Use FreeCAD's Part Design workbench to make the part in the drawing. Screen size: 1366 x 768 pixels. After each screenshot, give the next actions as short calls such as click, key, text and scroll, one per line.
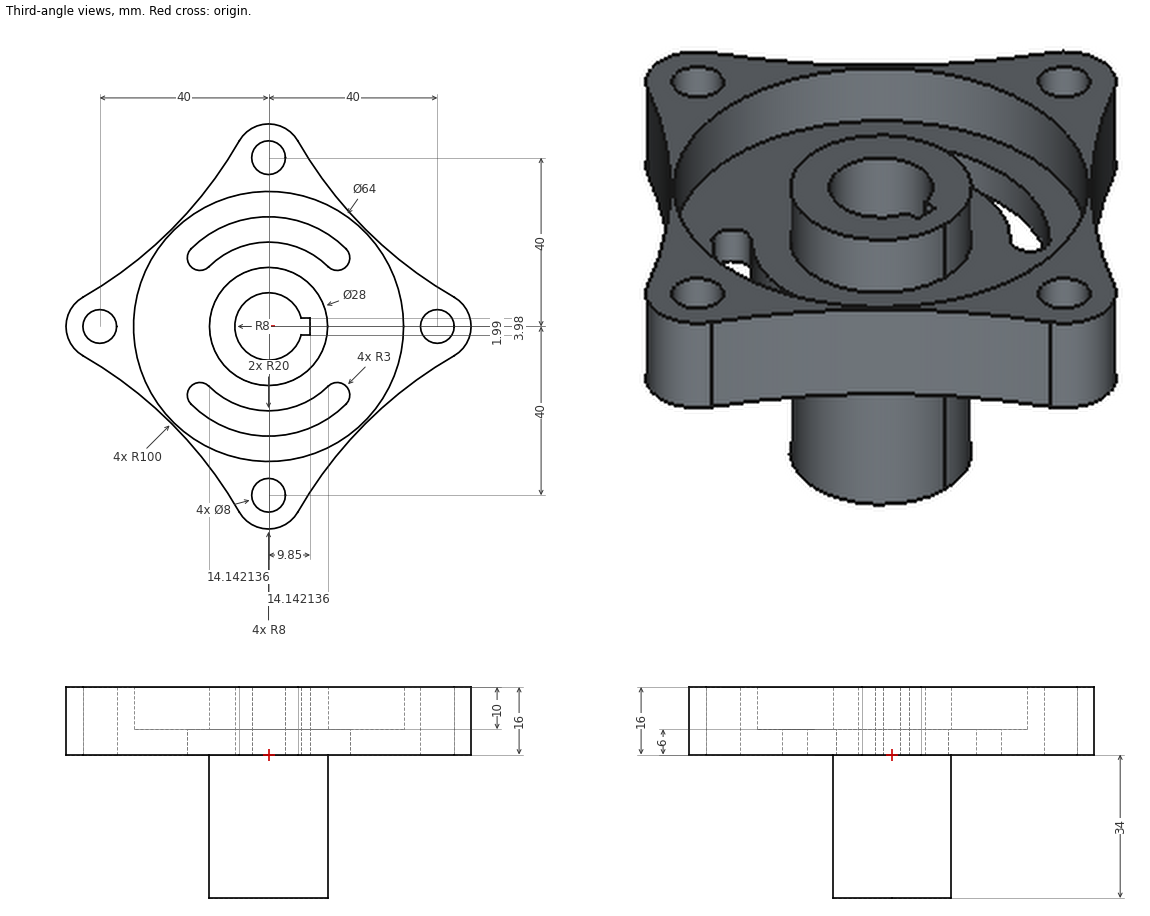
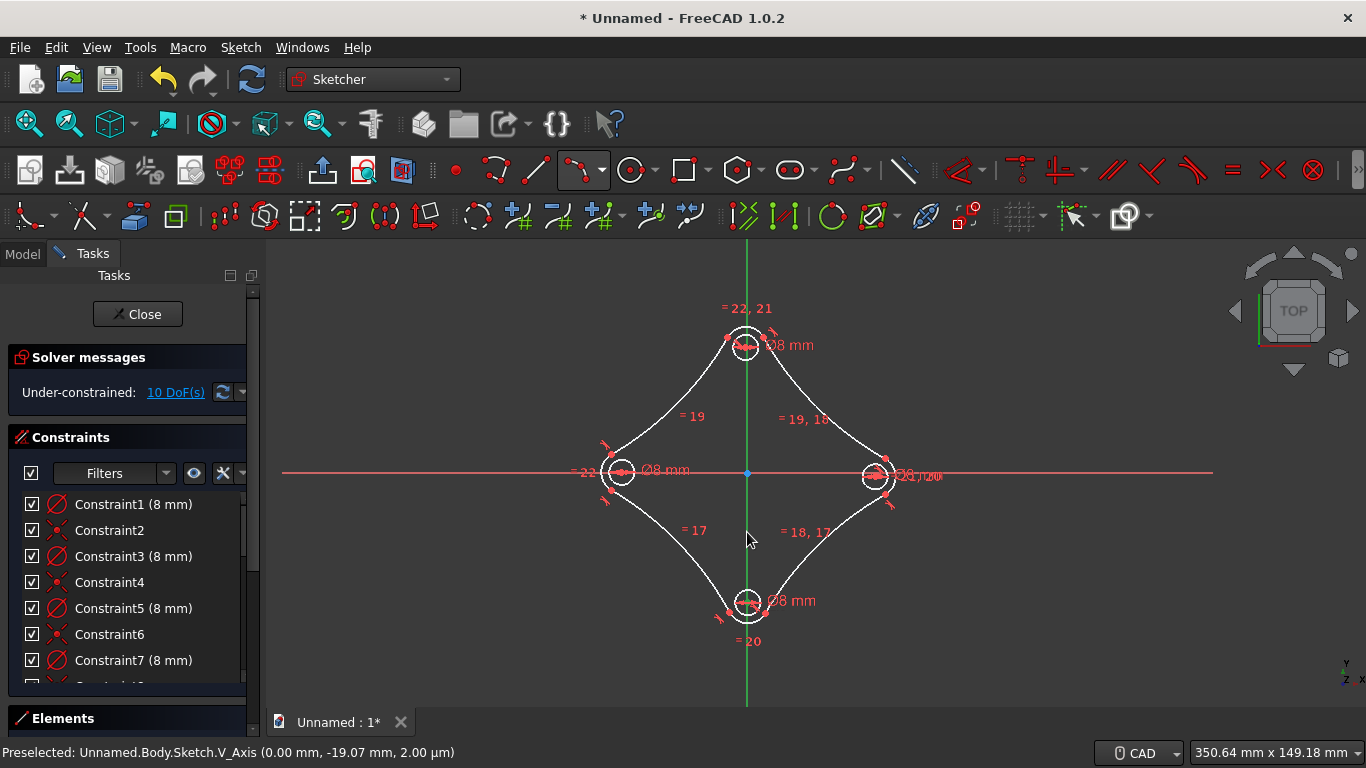
click(1020, 170)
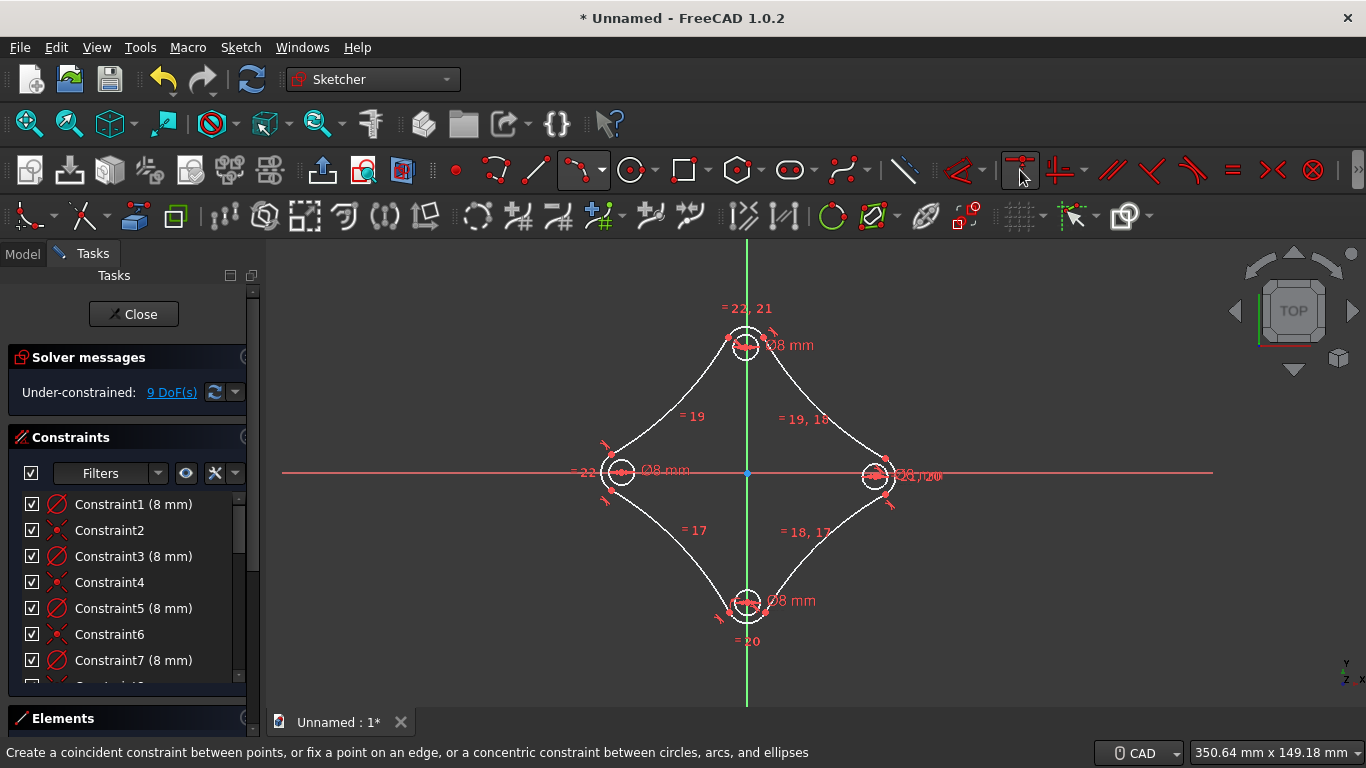
click(875, 477)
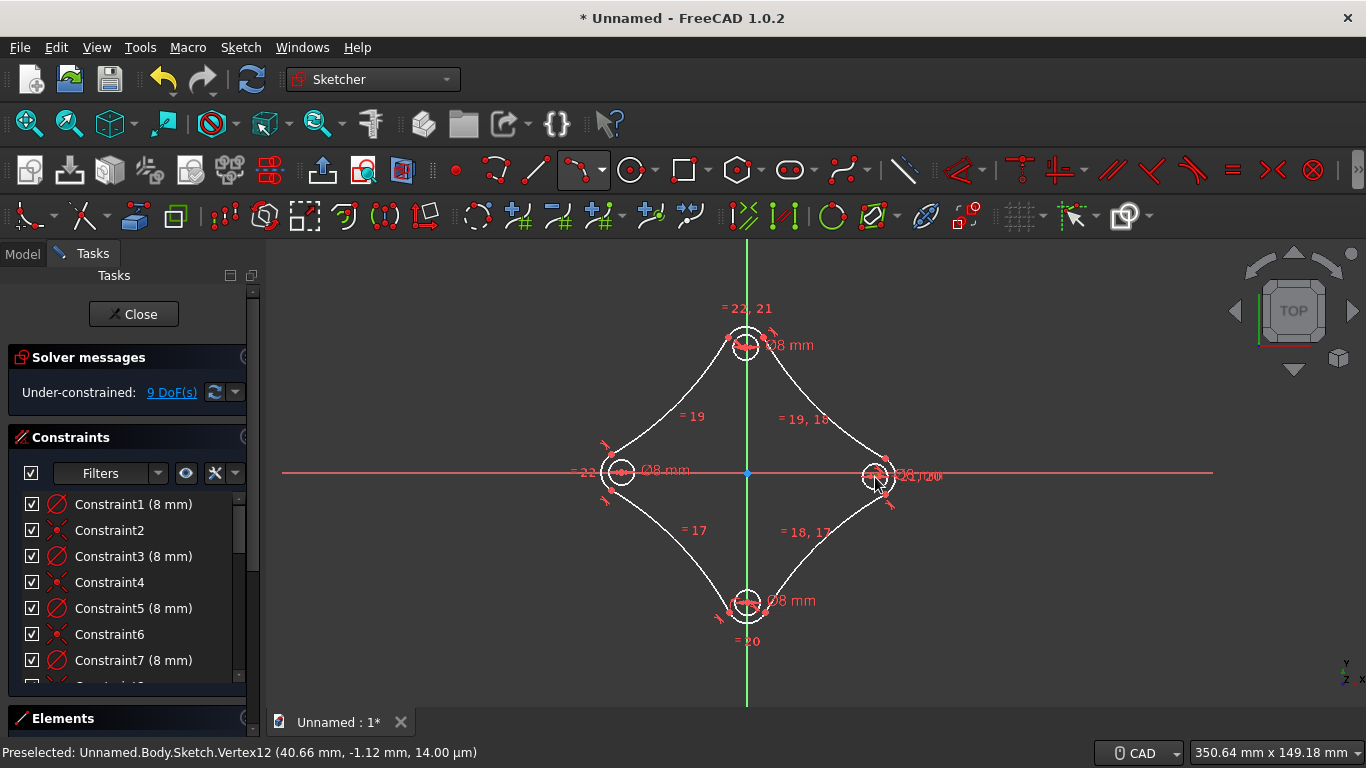
click(359, 473)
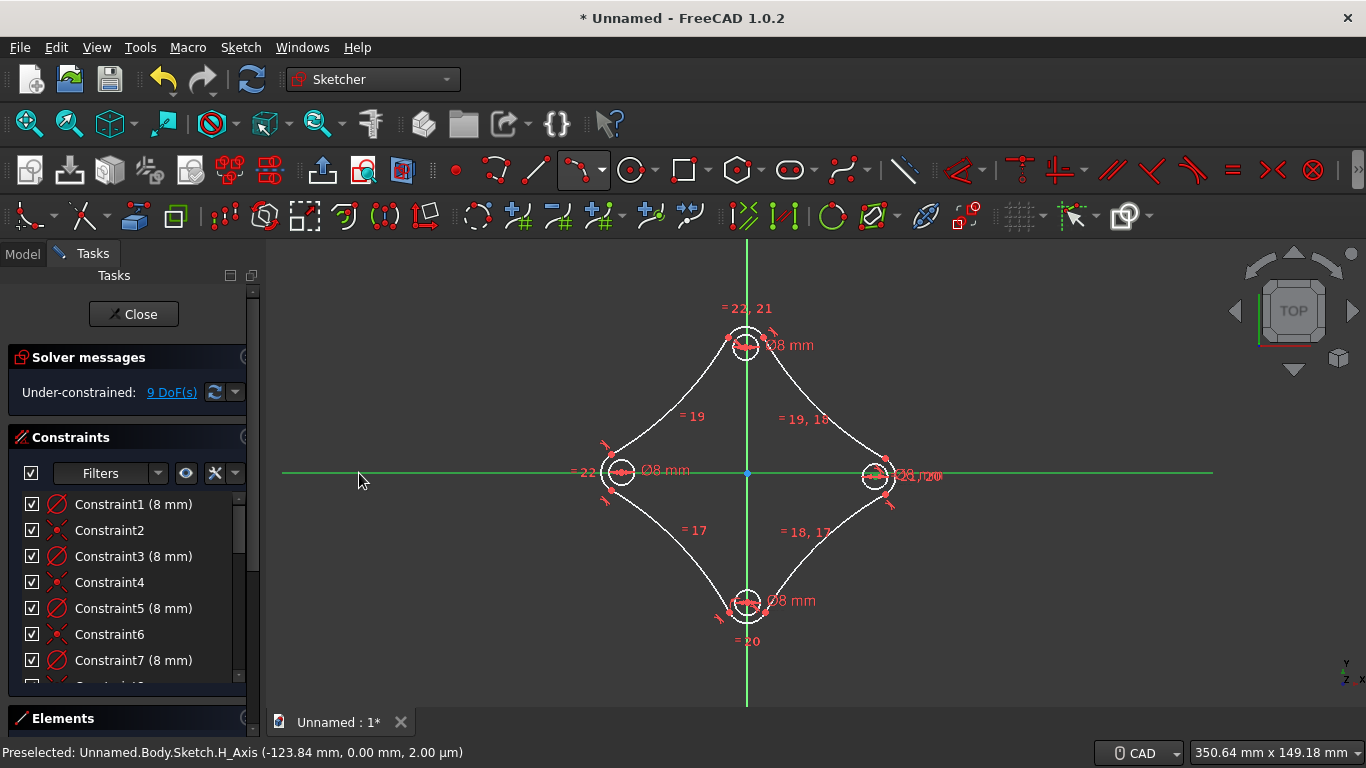
click(1020, 170)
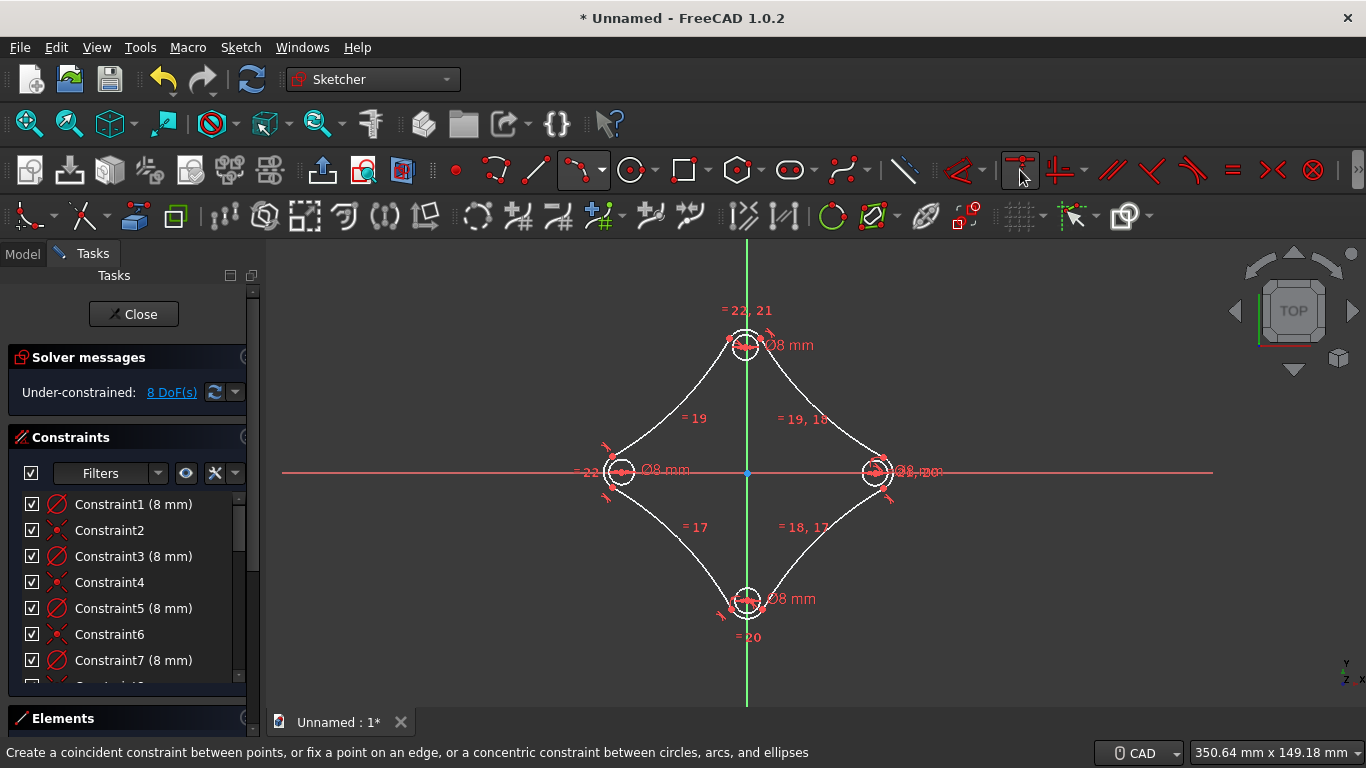
click(745, 347)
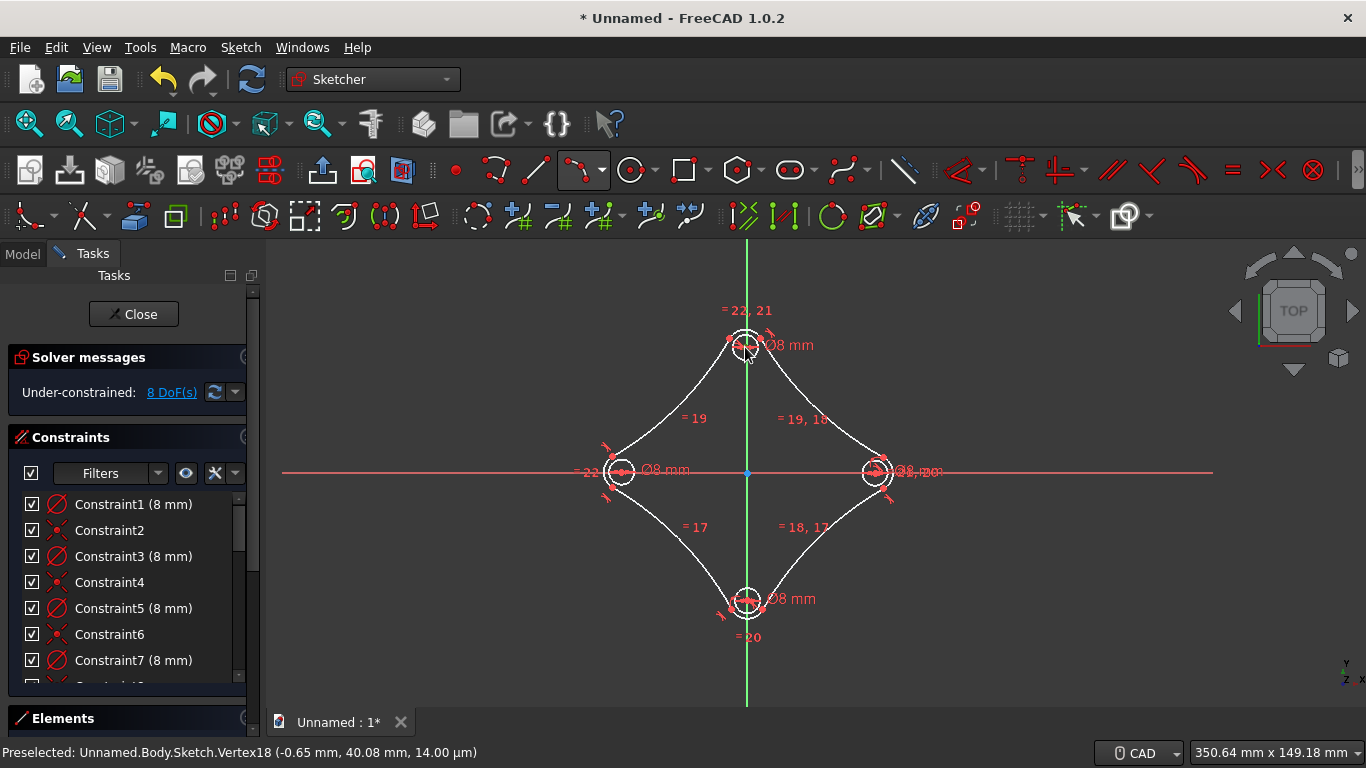
click(747, 650)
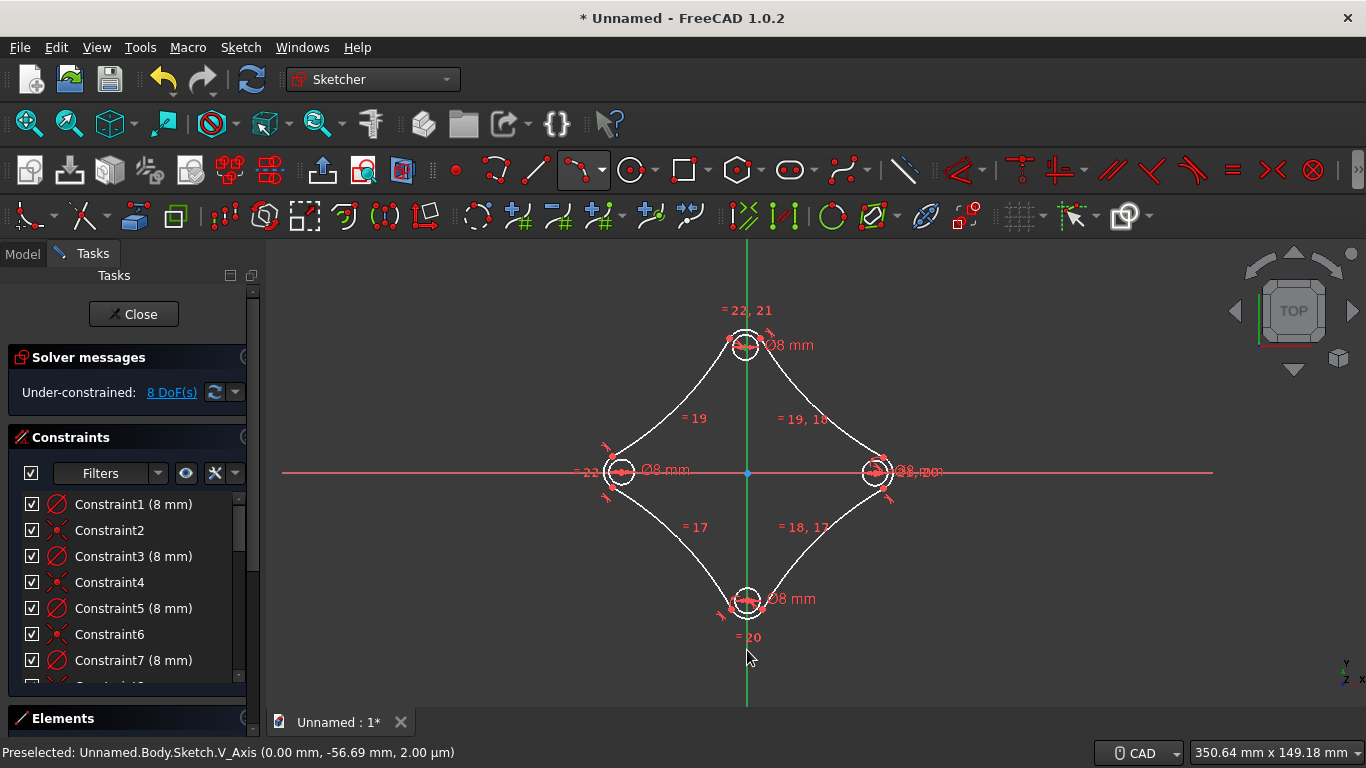
click(1020, 170)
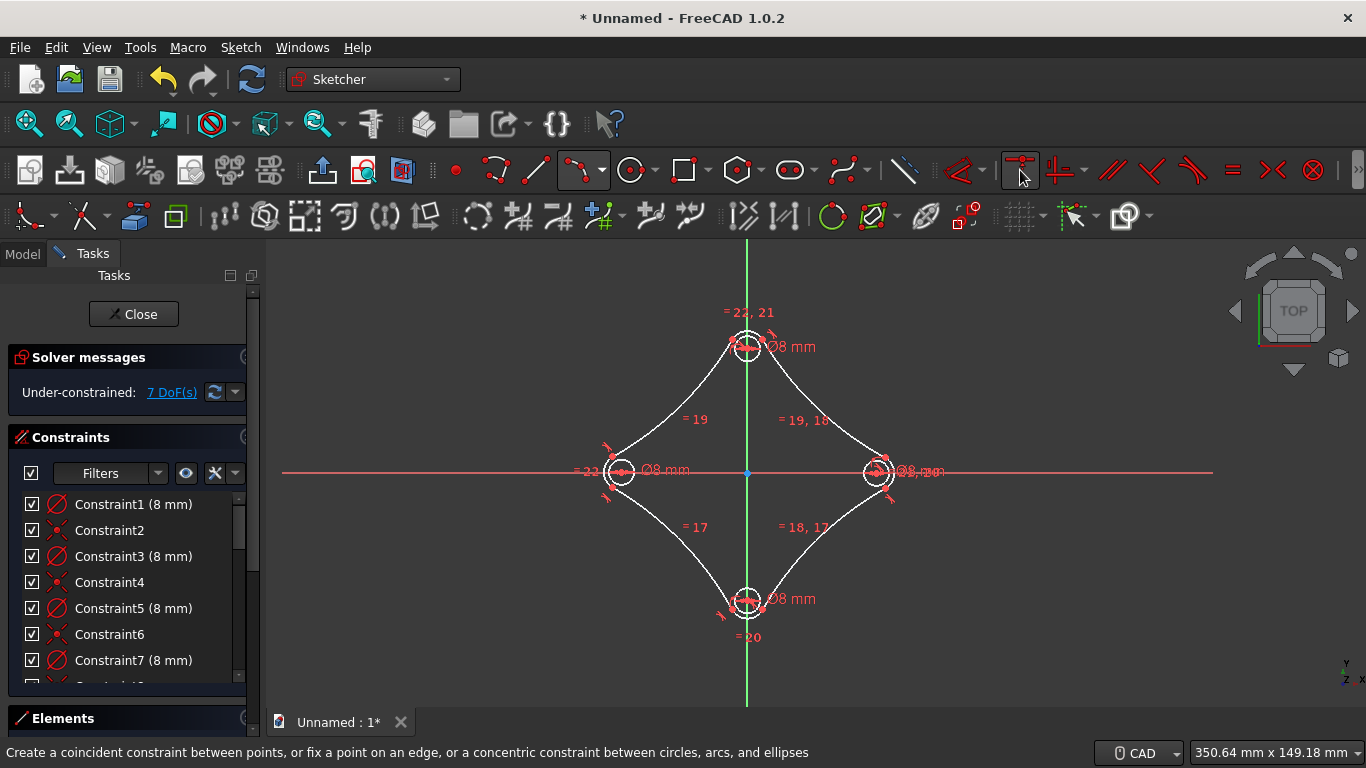
click(622, 472)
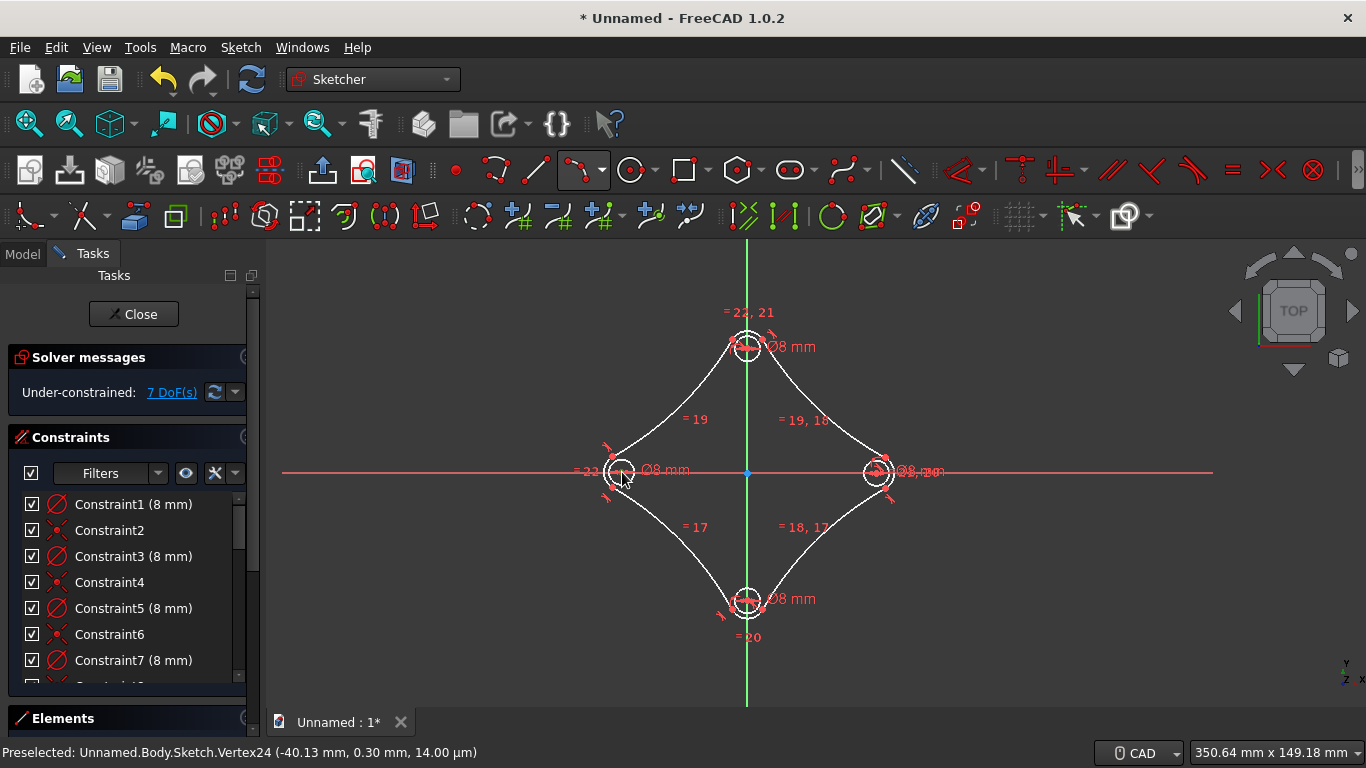
click(359, 473)